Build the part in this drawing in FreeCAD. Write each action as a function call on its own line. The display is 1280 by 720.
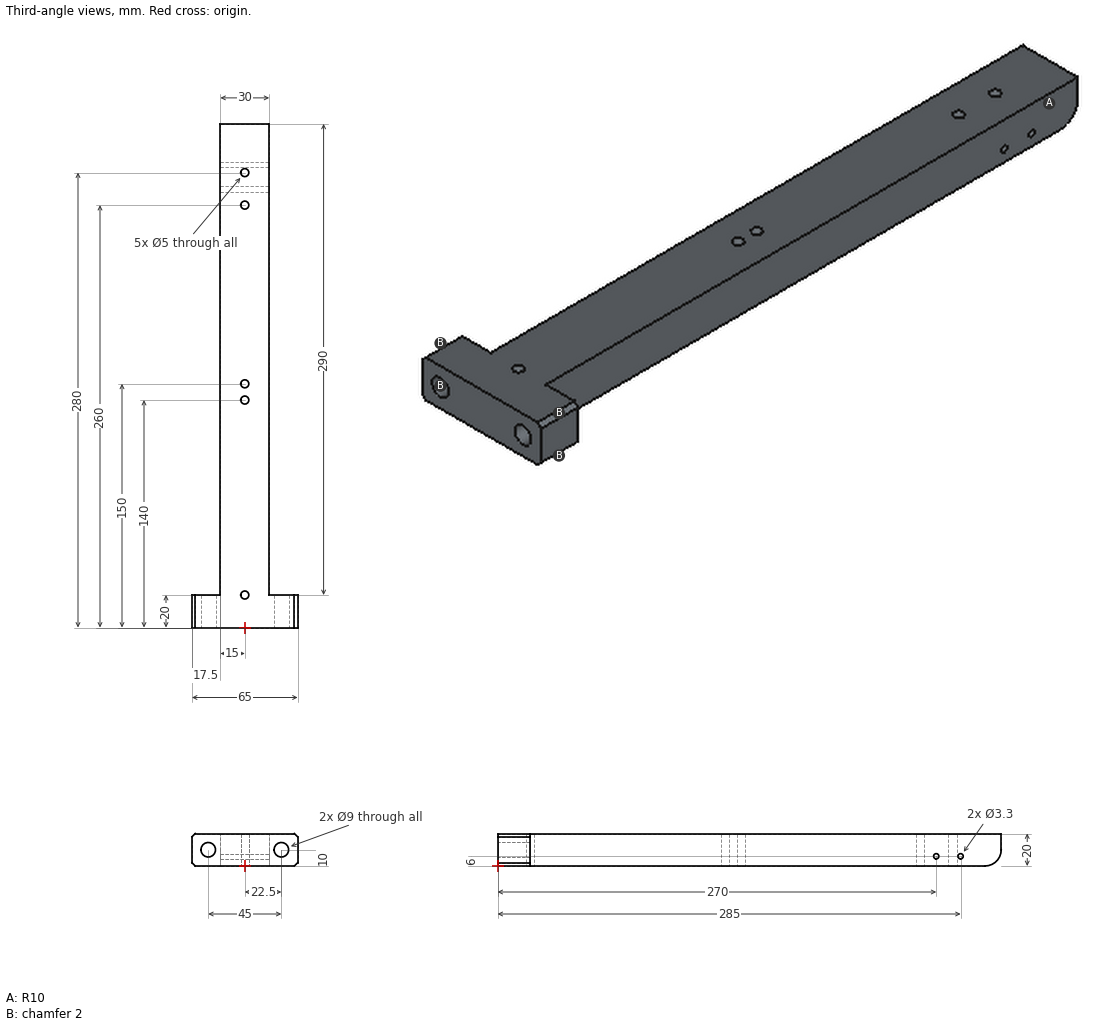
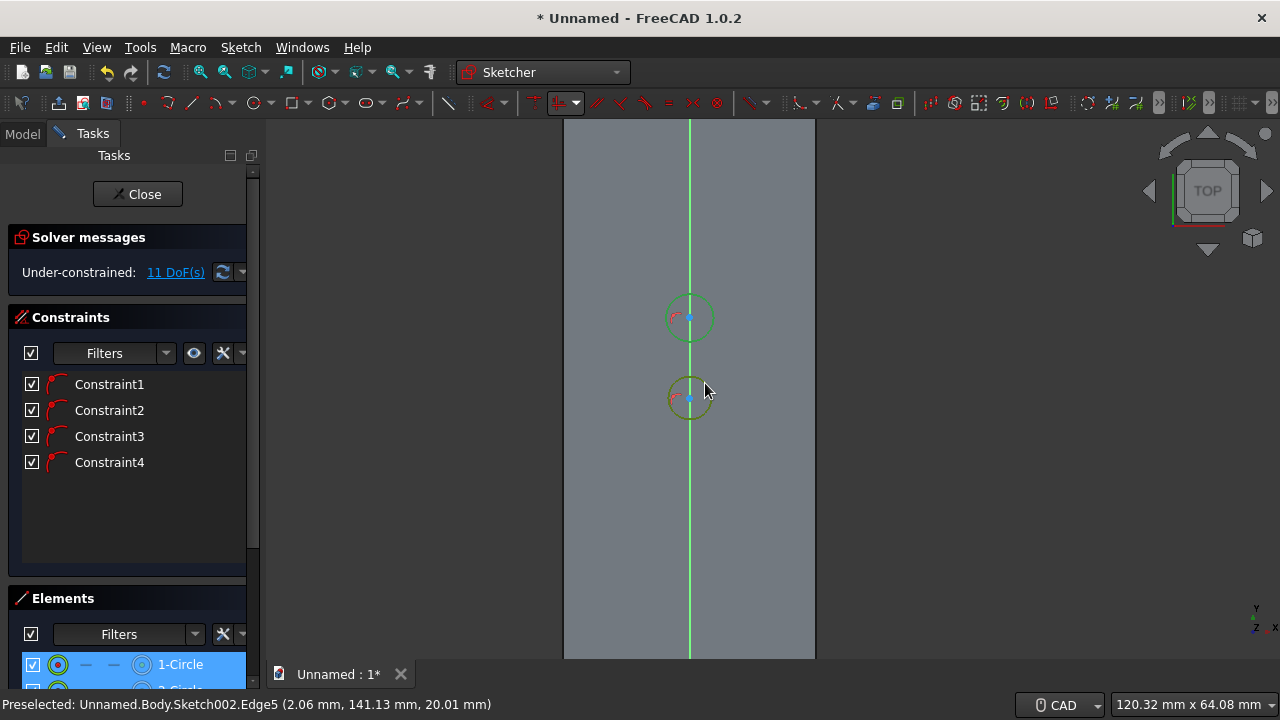
click(670, 104)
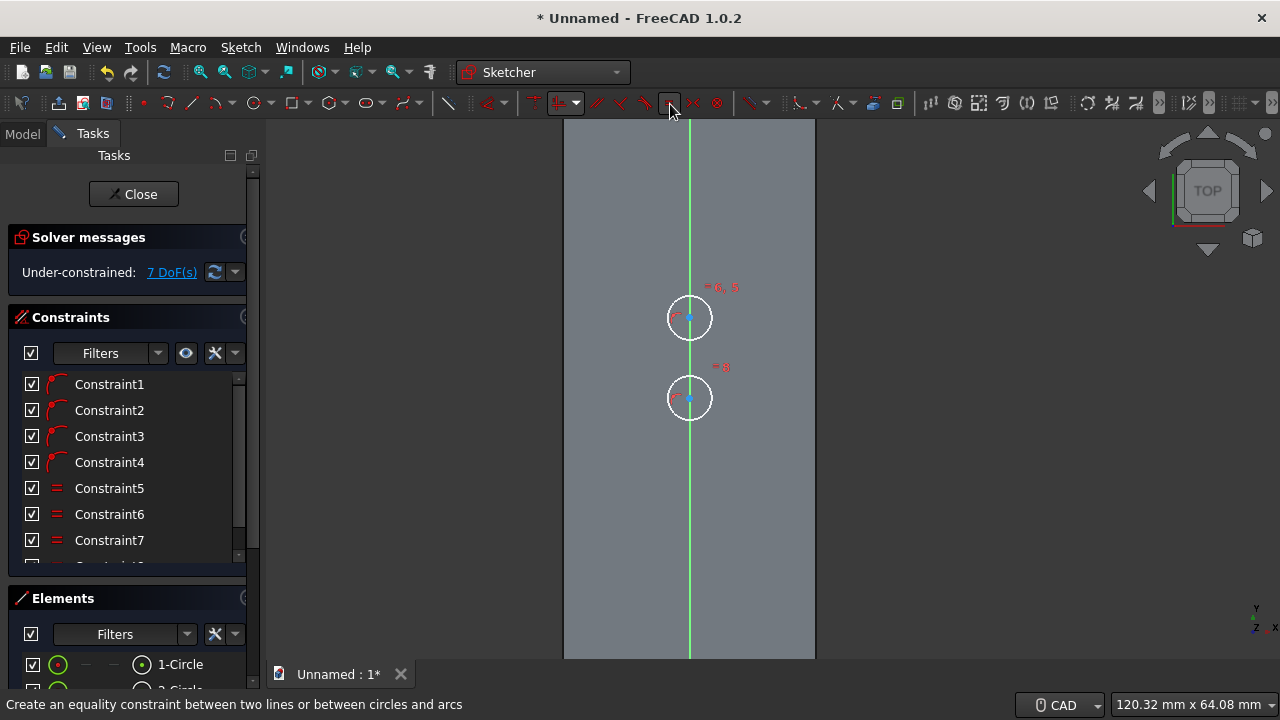
scroll(707, 390, down, 10)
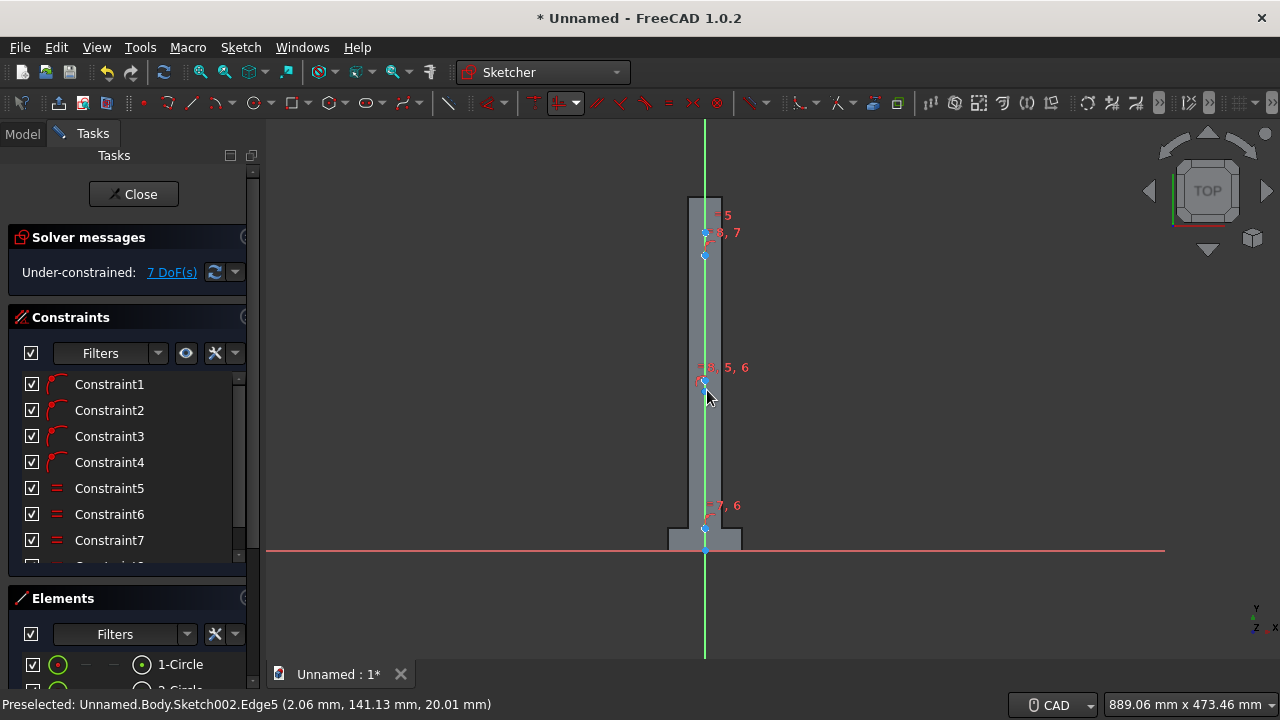
click(706, 233)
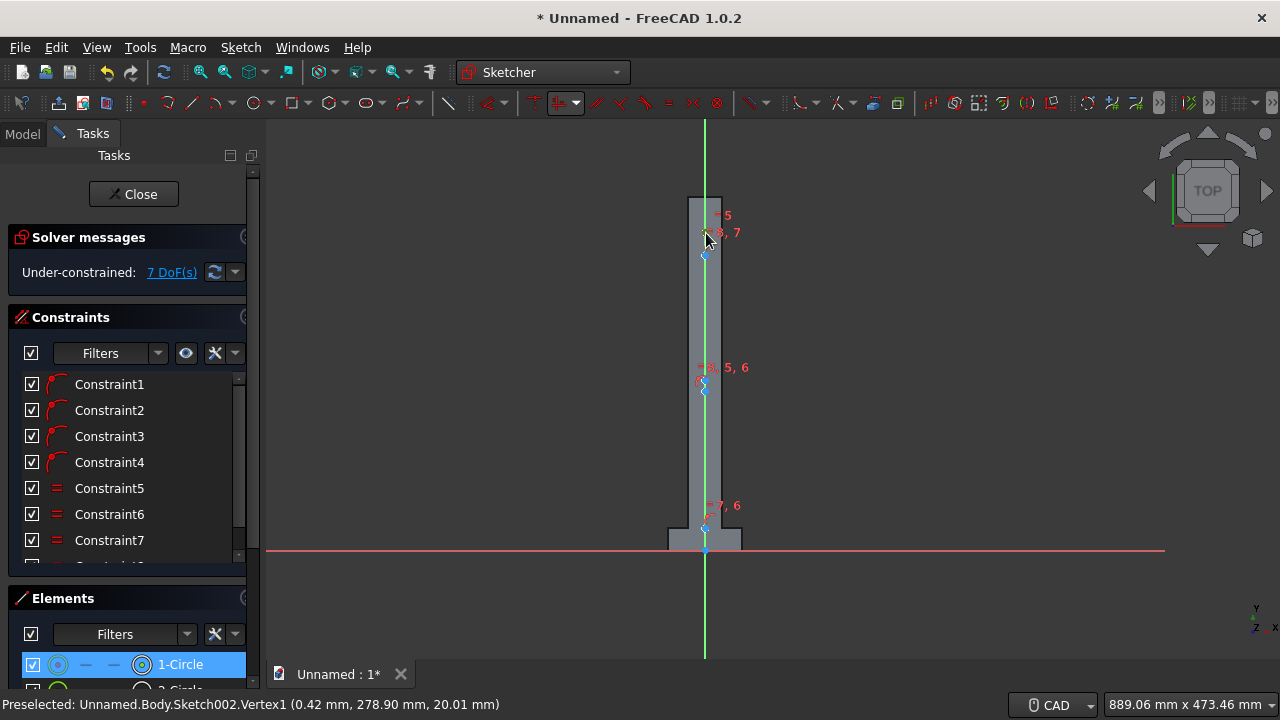
click(705, 596)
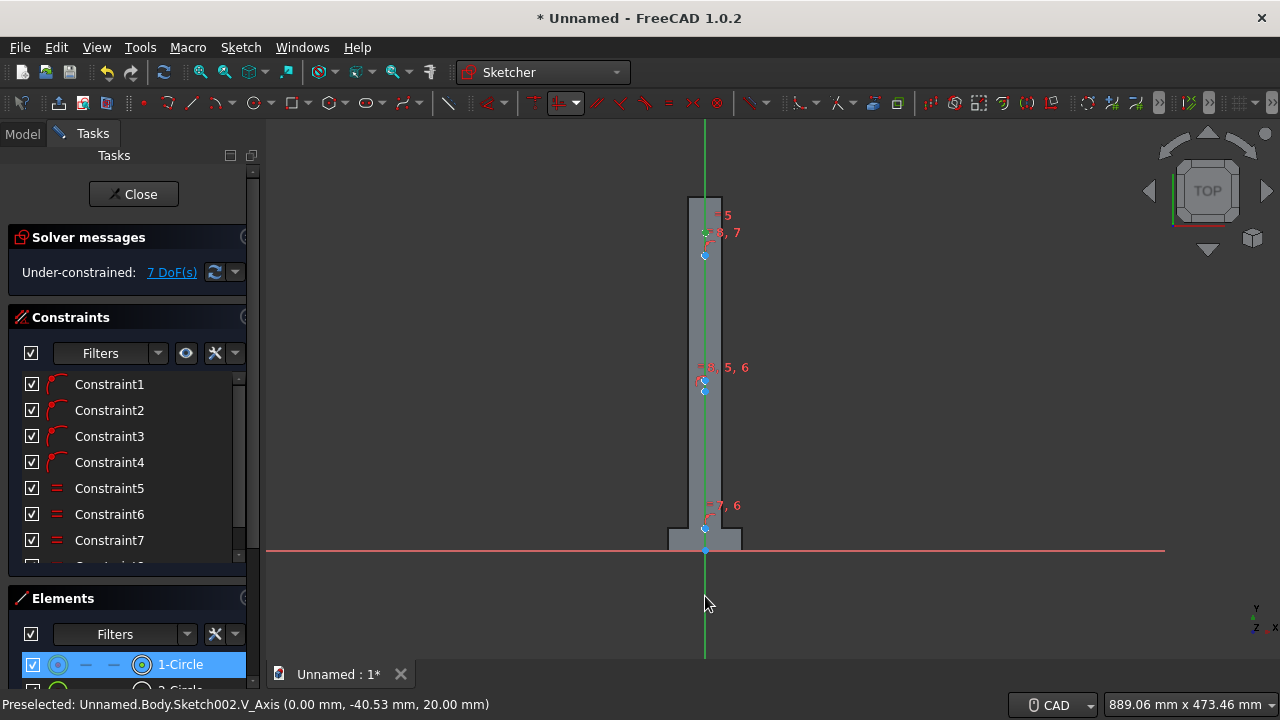
click(534, 104)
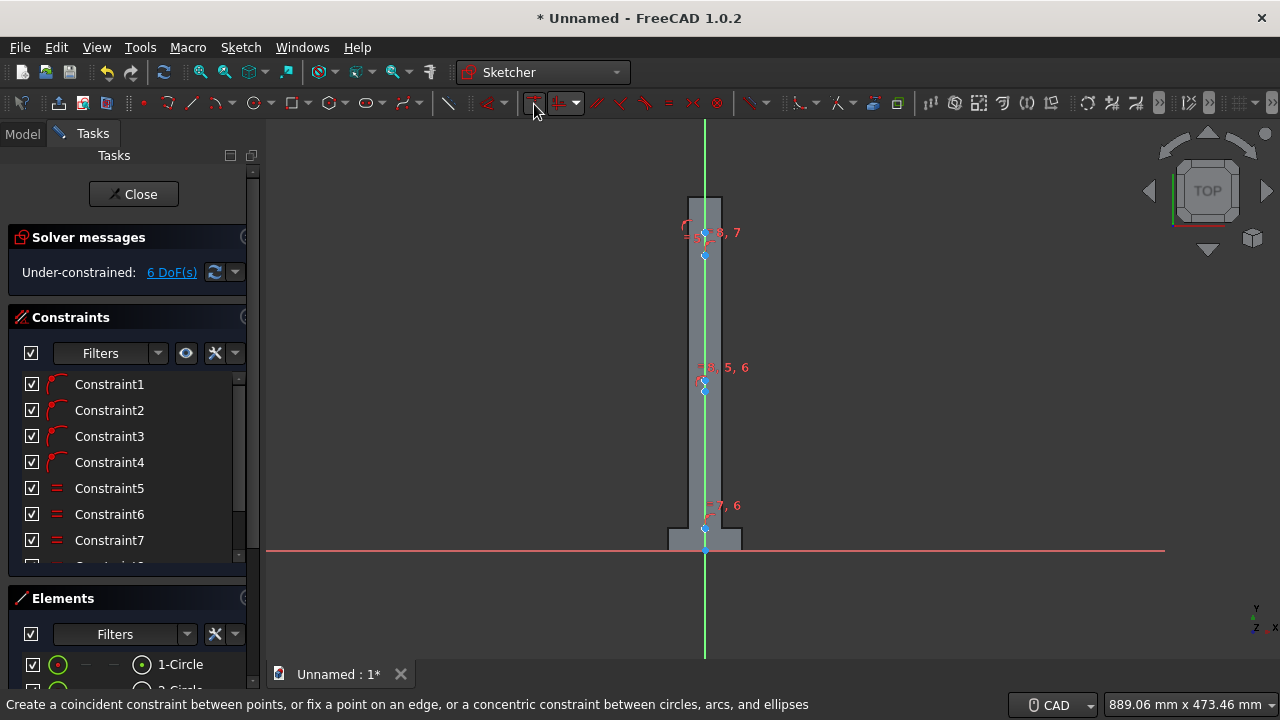
click(488, 104)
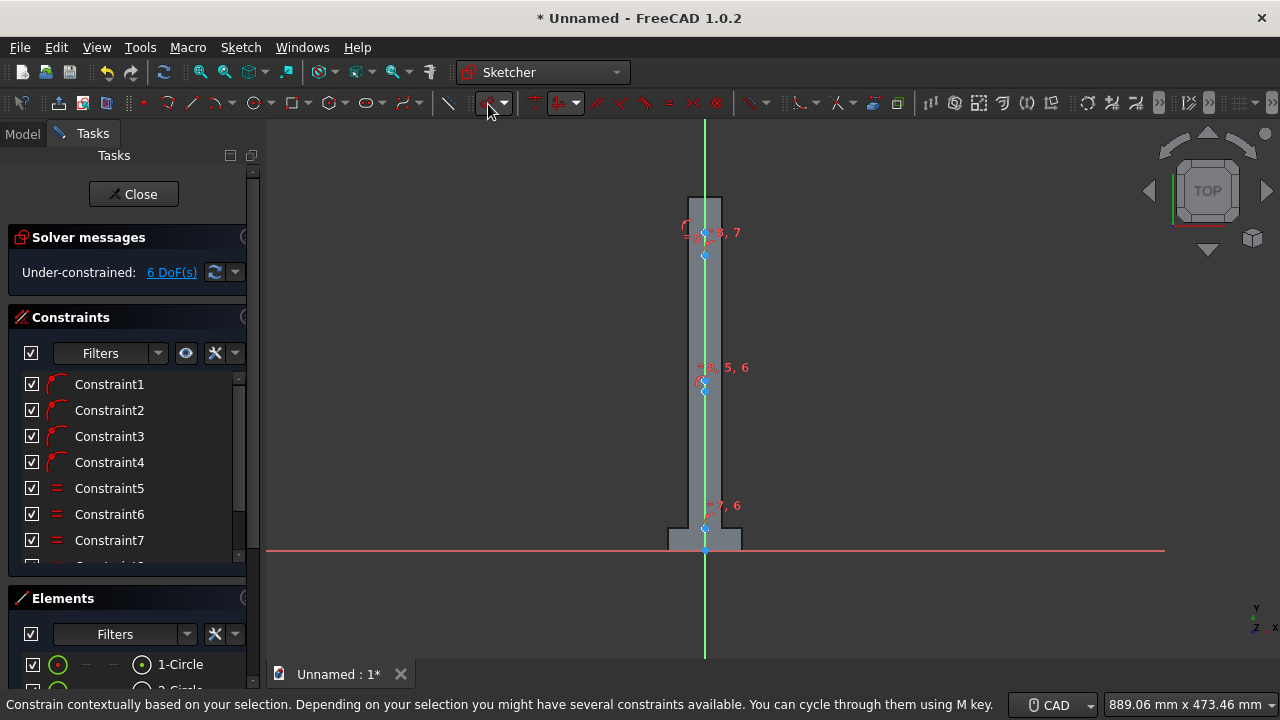
scroll(702, 233, up, 10)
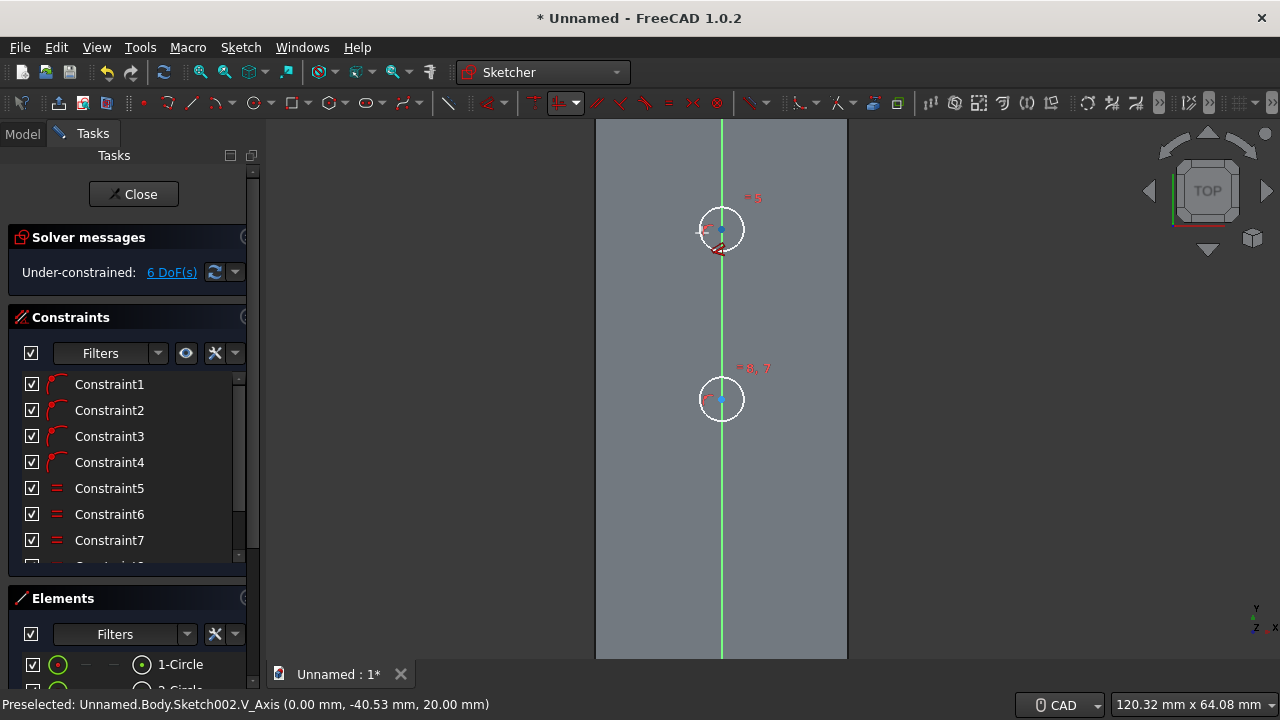
click(700, 229)
click(668, 229)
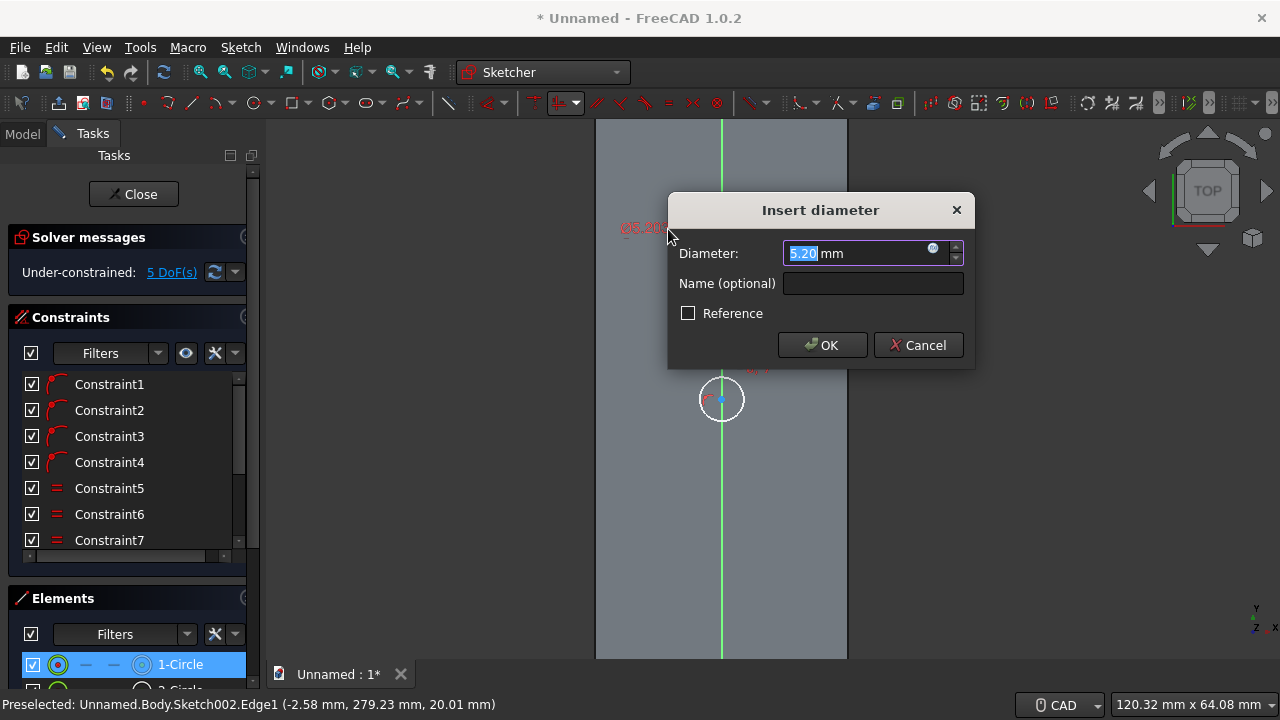
text(5)
key(Return)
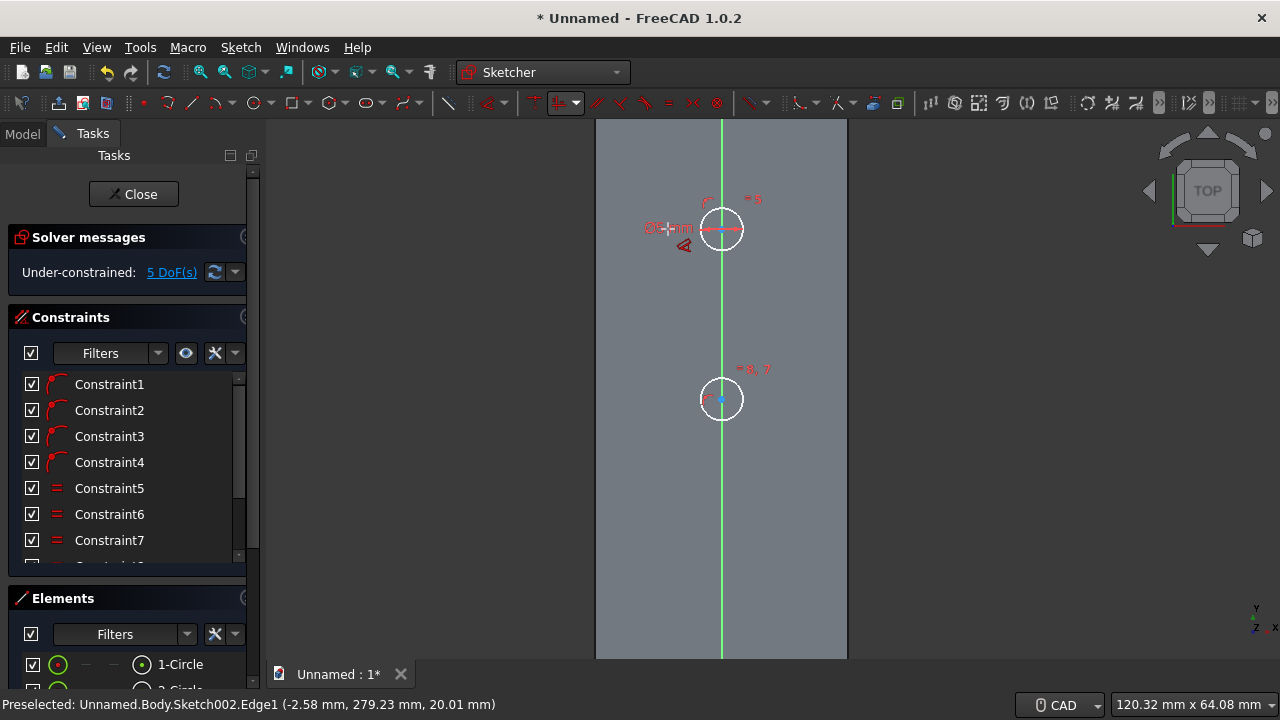
scroll(702, 232, down, 10)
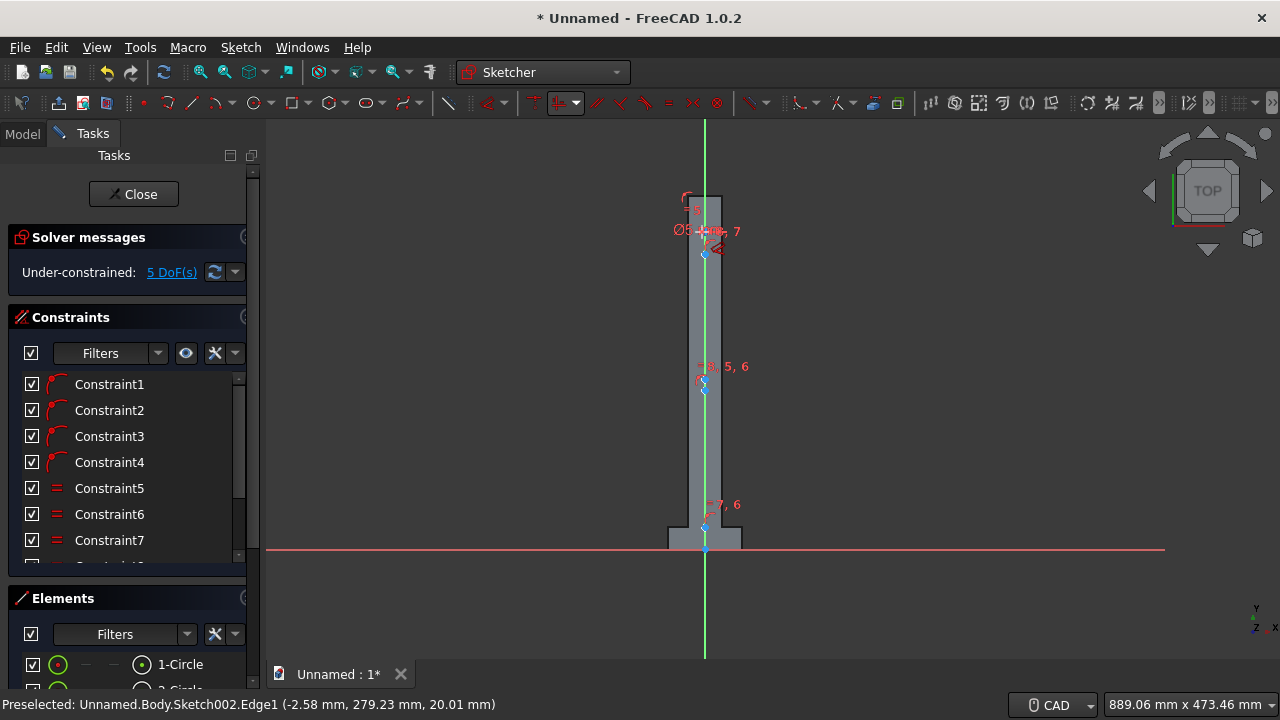
scroll(705, 528, up, 3)